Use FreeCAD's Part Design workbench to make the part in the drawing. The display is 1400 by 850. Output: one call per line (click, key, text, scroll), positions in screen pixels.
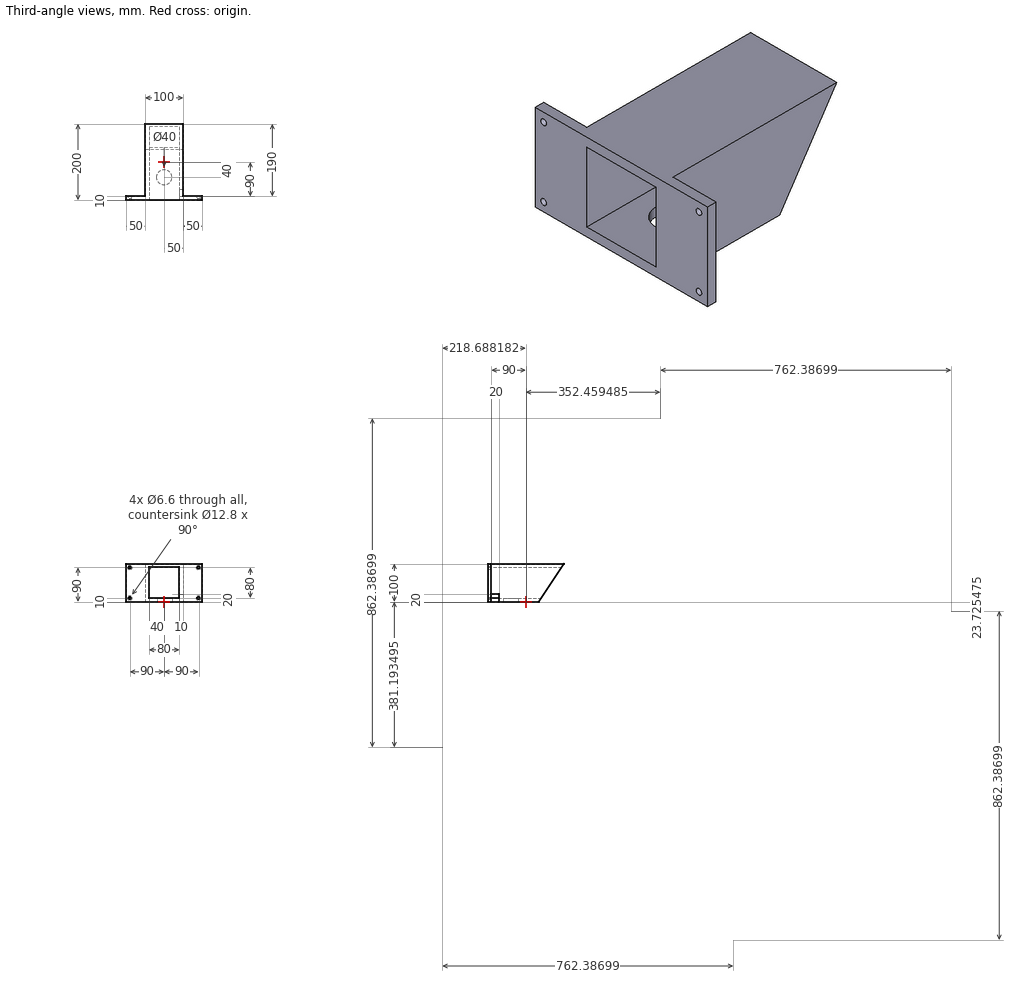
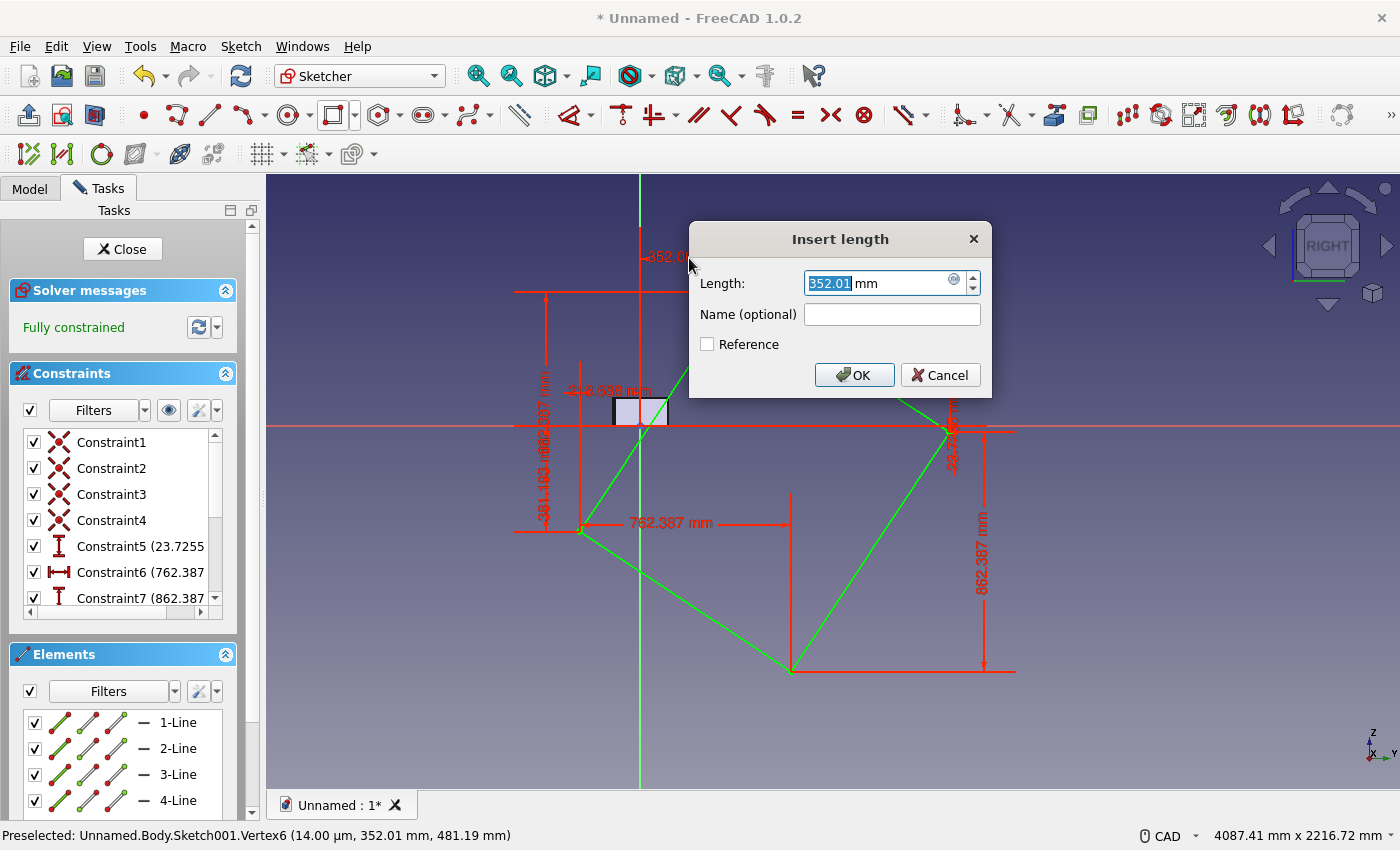
text(352.459485)
key(Return)
key(Escape)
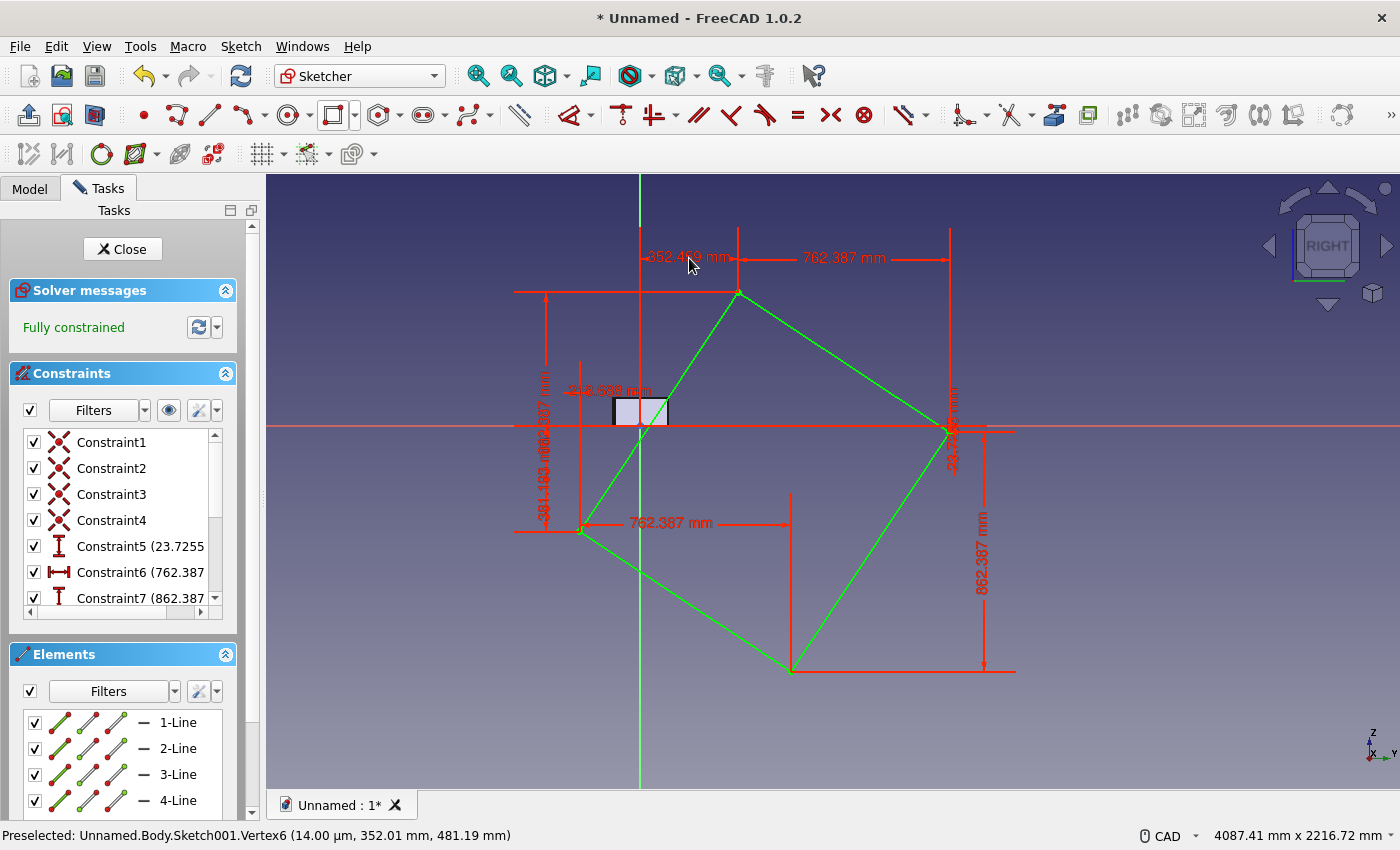
click(123, 249)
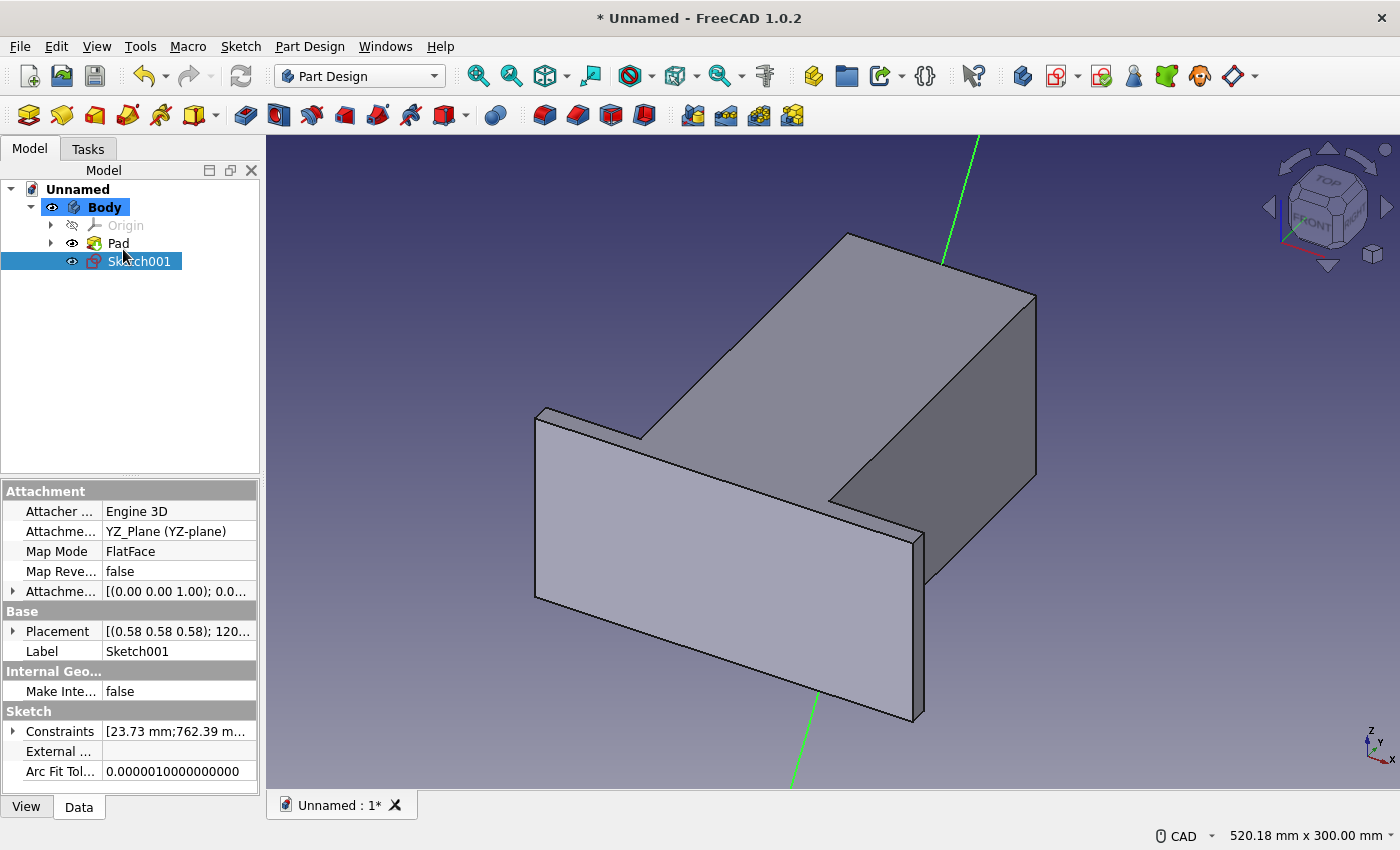
click(246, 116)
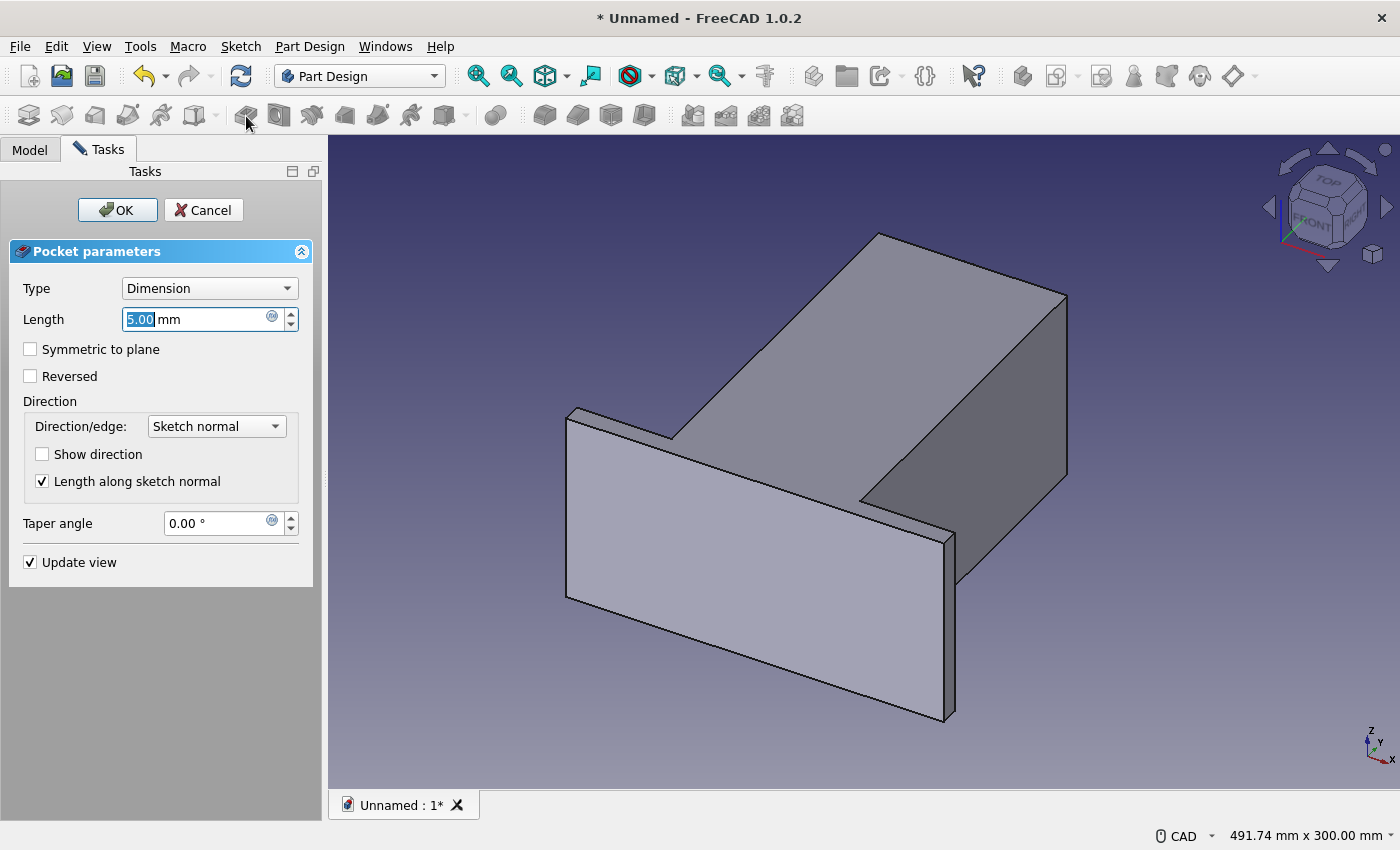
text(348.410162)
key(Tab)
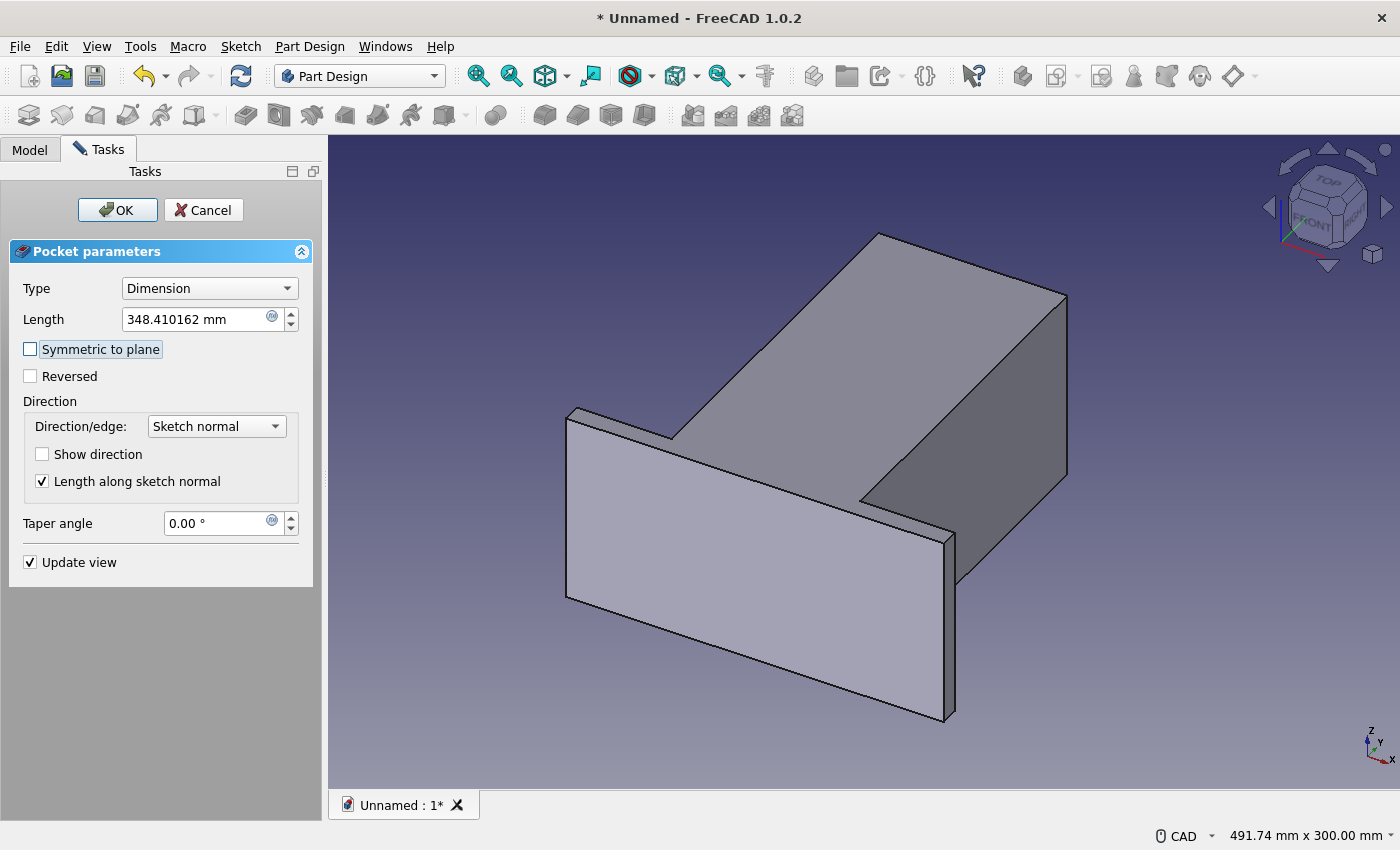
click(31, 349)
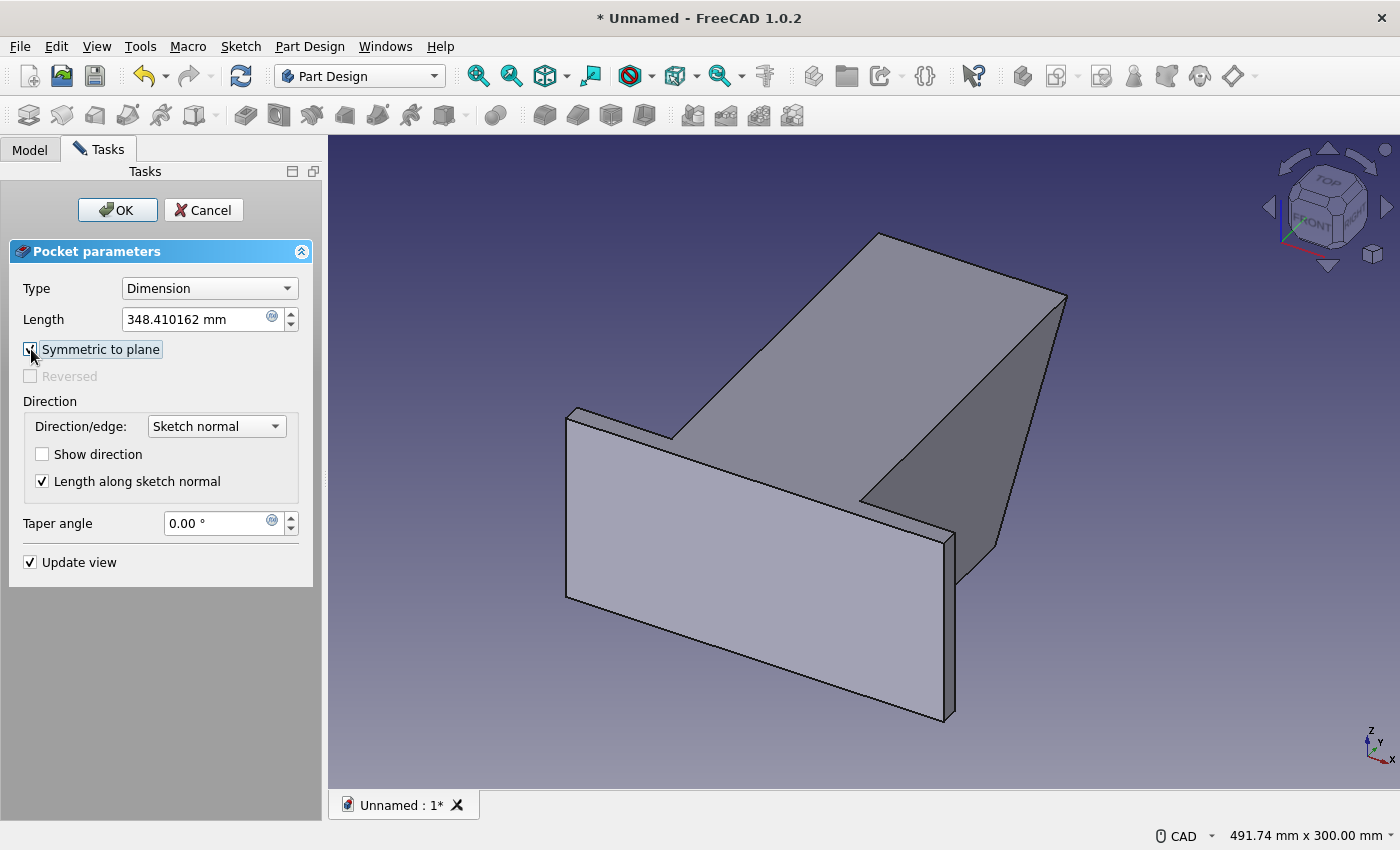
click(118, 210)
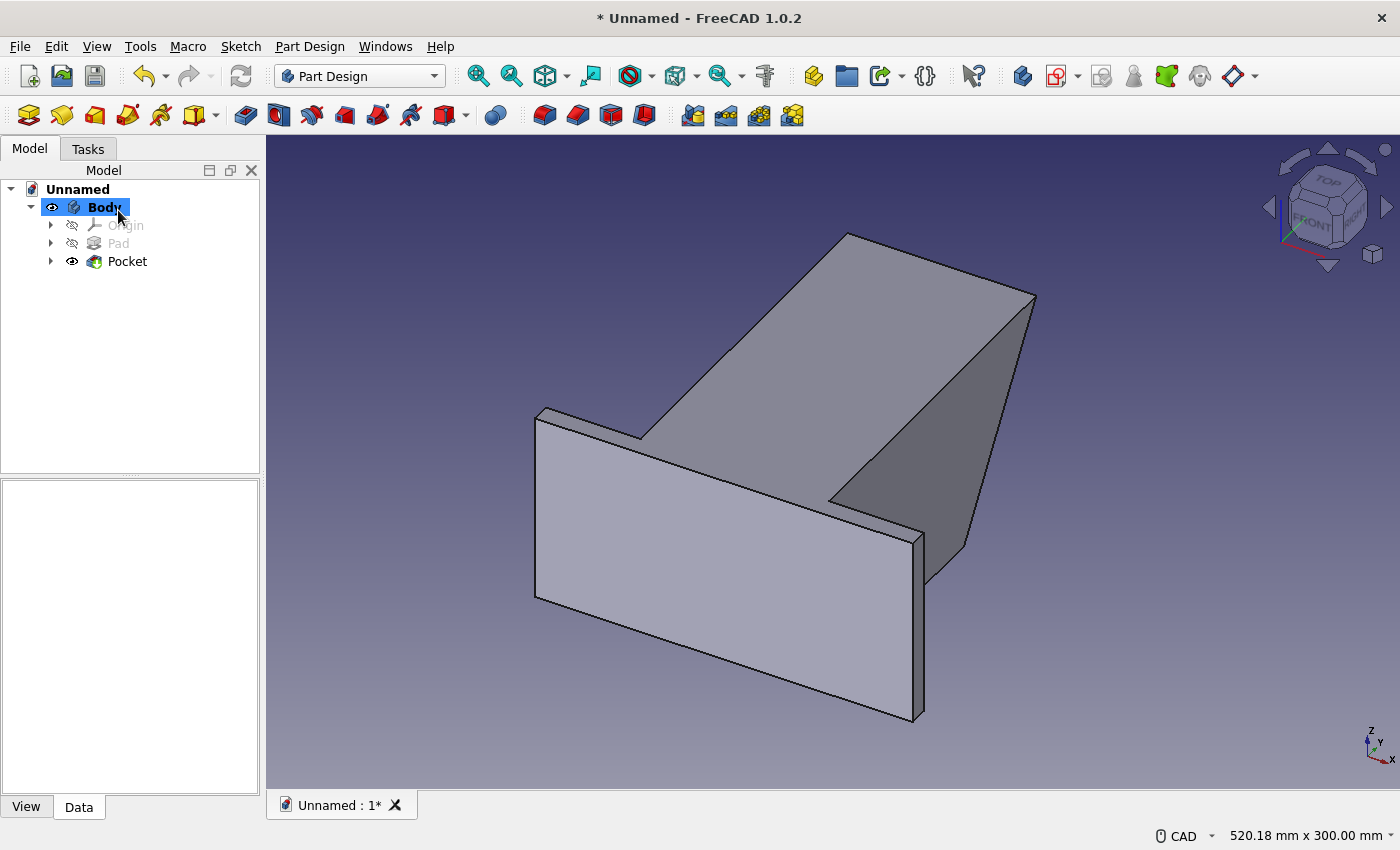
click(1056, 76)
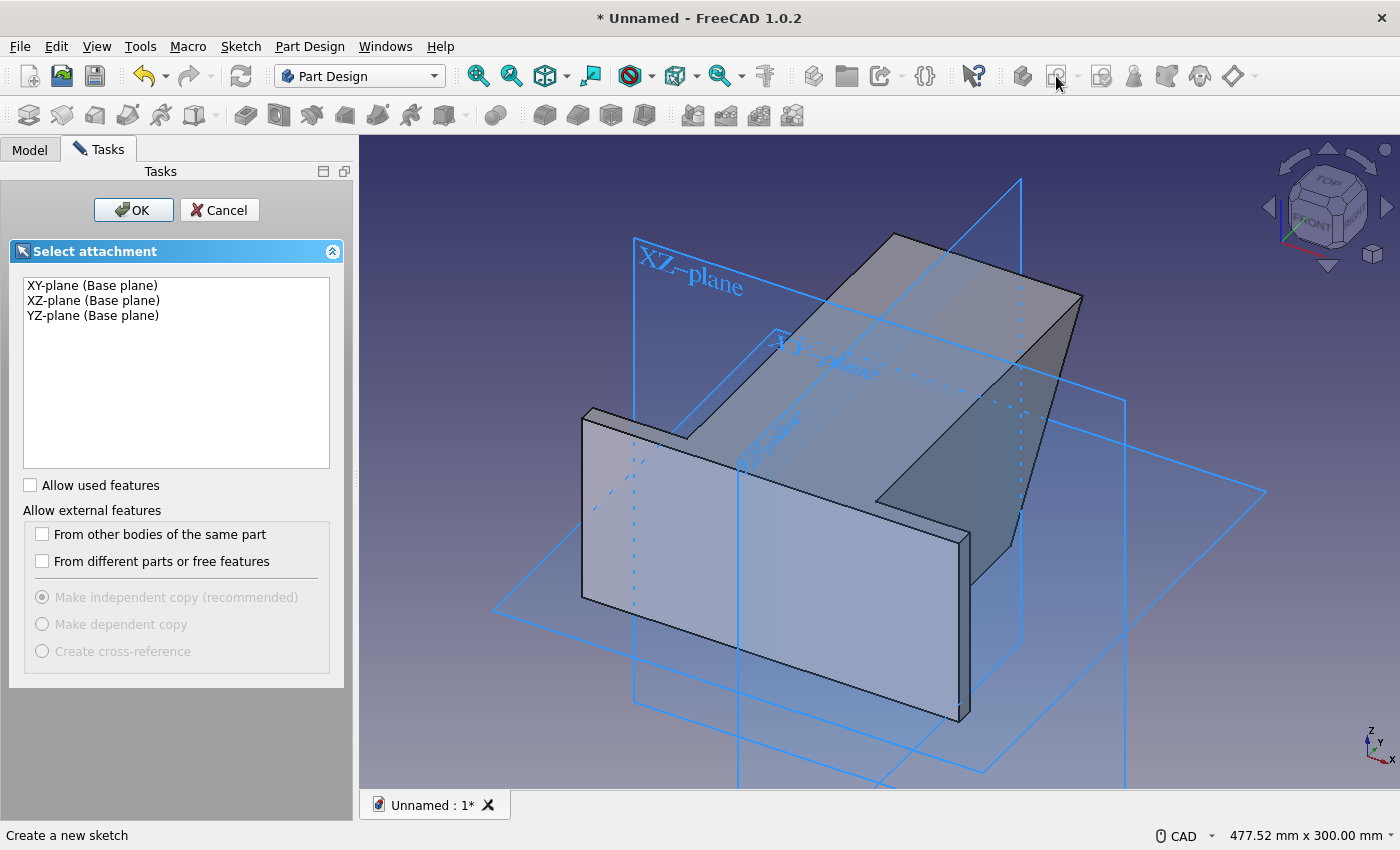
click(84, 300)